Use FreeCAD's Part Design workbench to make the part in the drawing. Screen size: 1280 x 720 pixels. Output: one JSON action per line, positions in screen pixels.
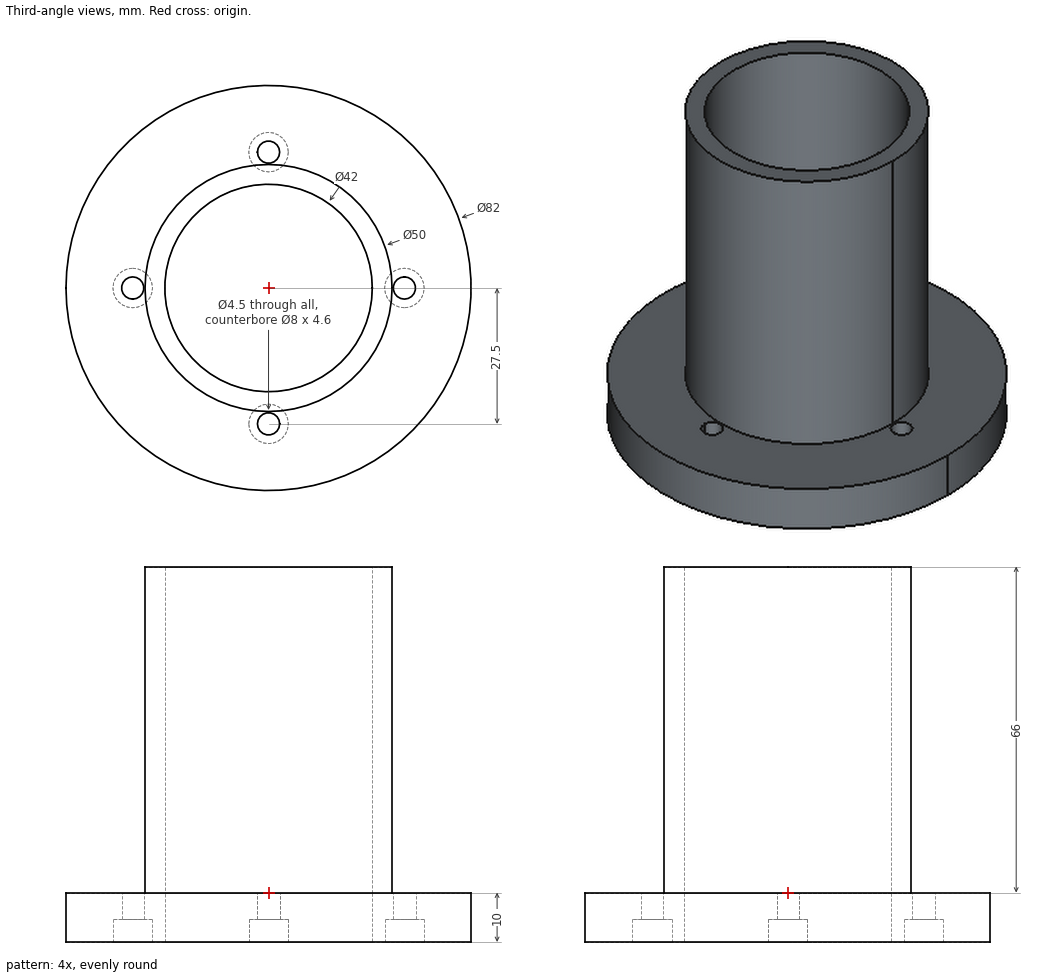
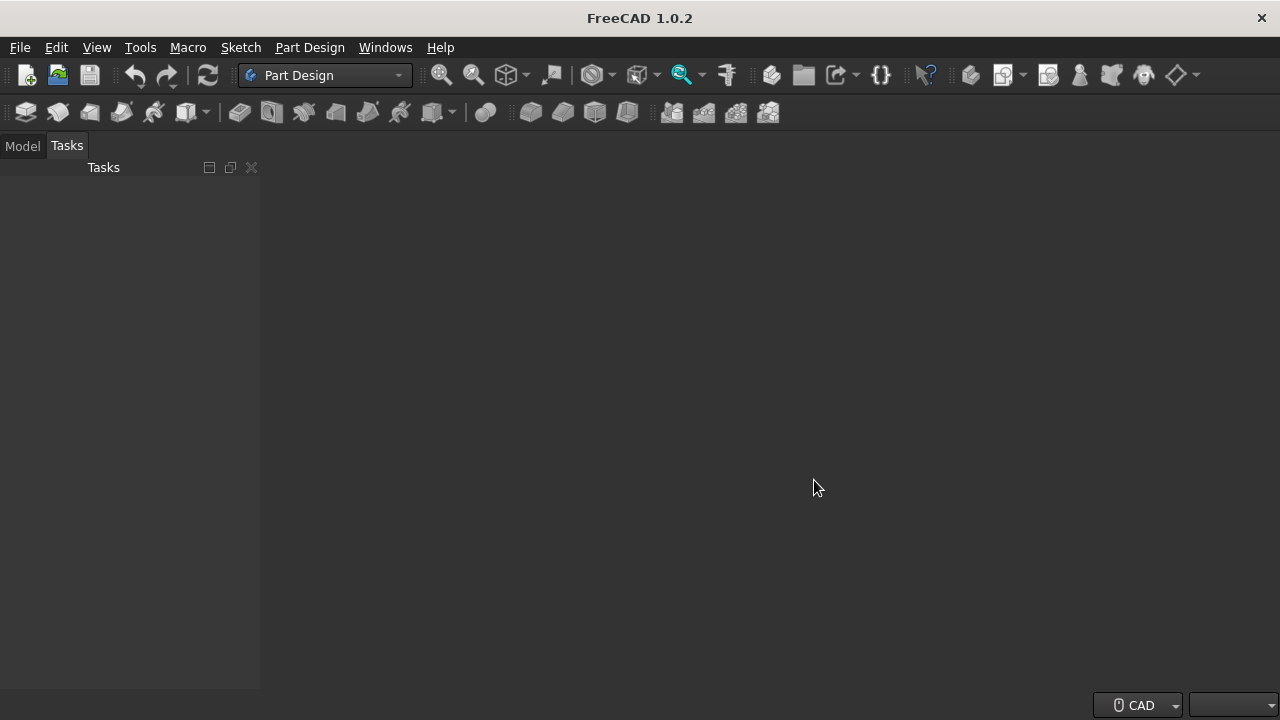
{"action": "left_click", "coordinate": [26, 76]}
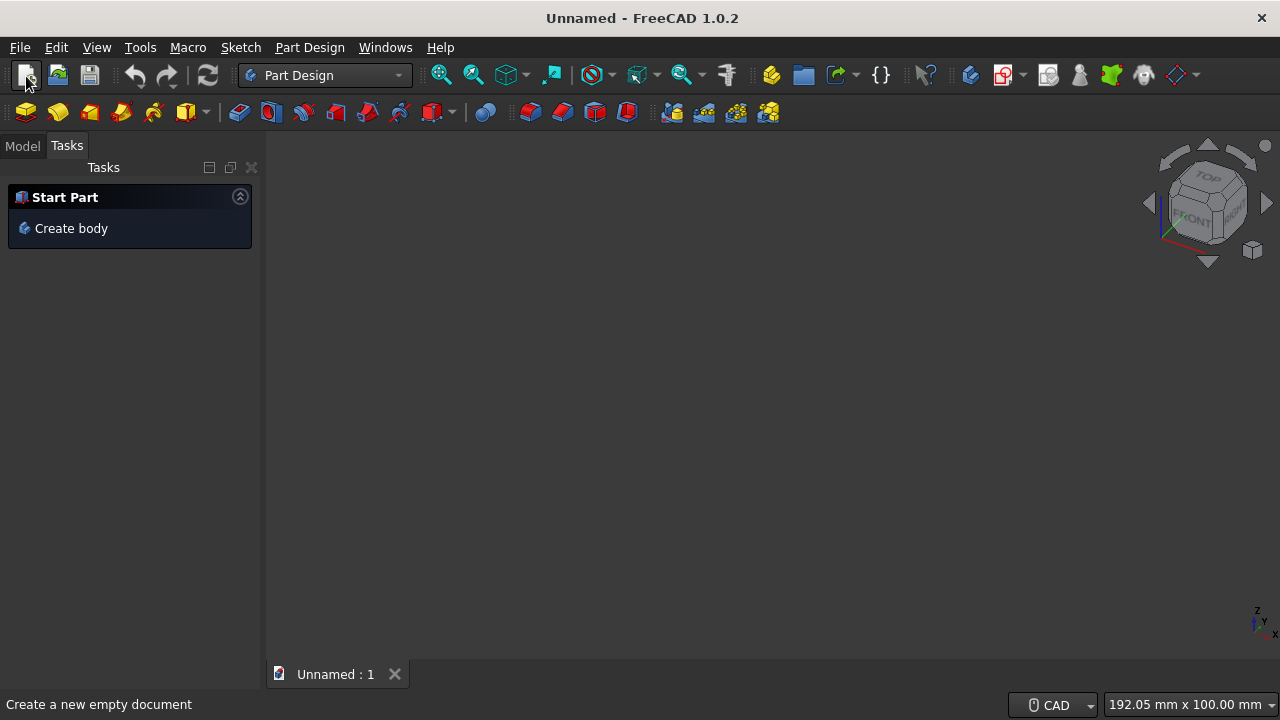
{"action": "left_click", "coordinate": [1004, 76]}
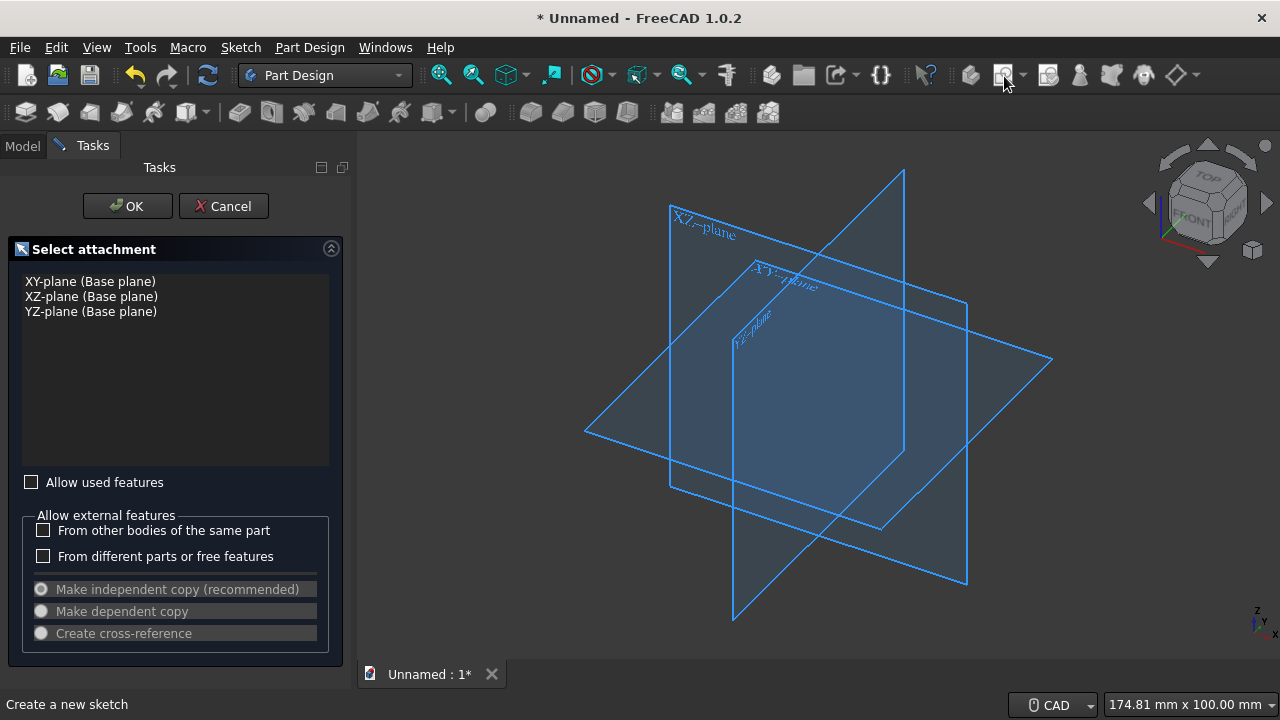
{"action": "left_click", "coordinate": [82, 282]}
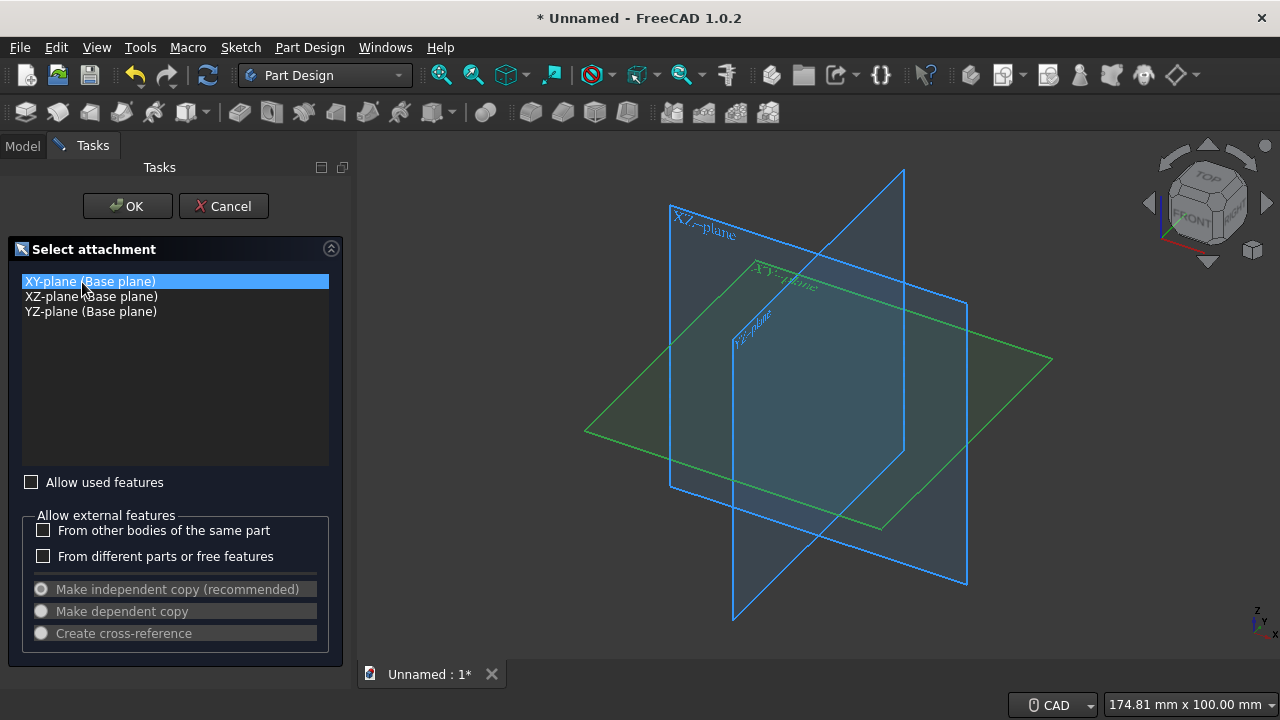
{"action": "left_click", "coordinate": [128, 206]}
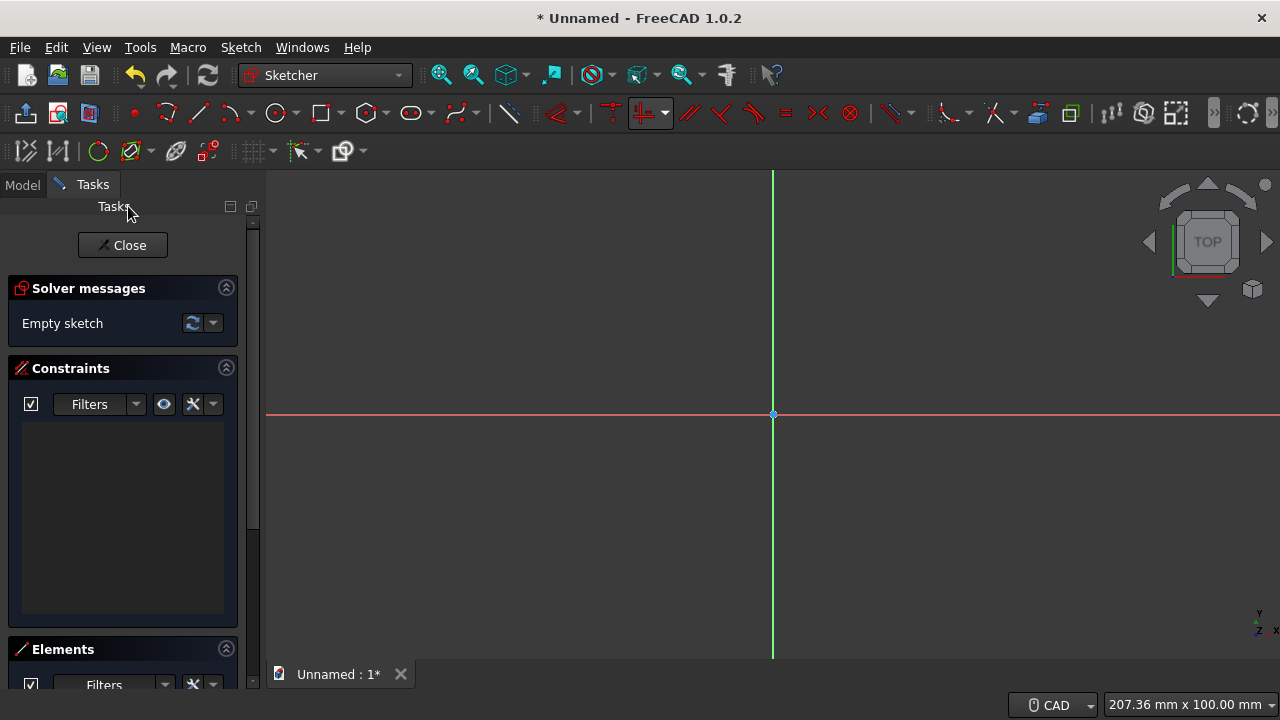
{"action": "key", "text": "g c"}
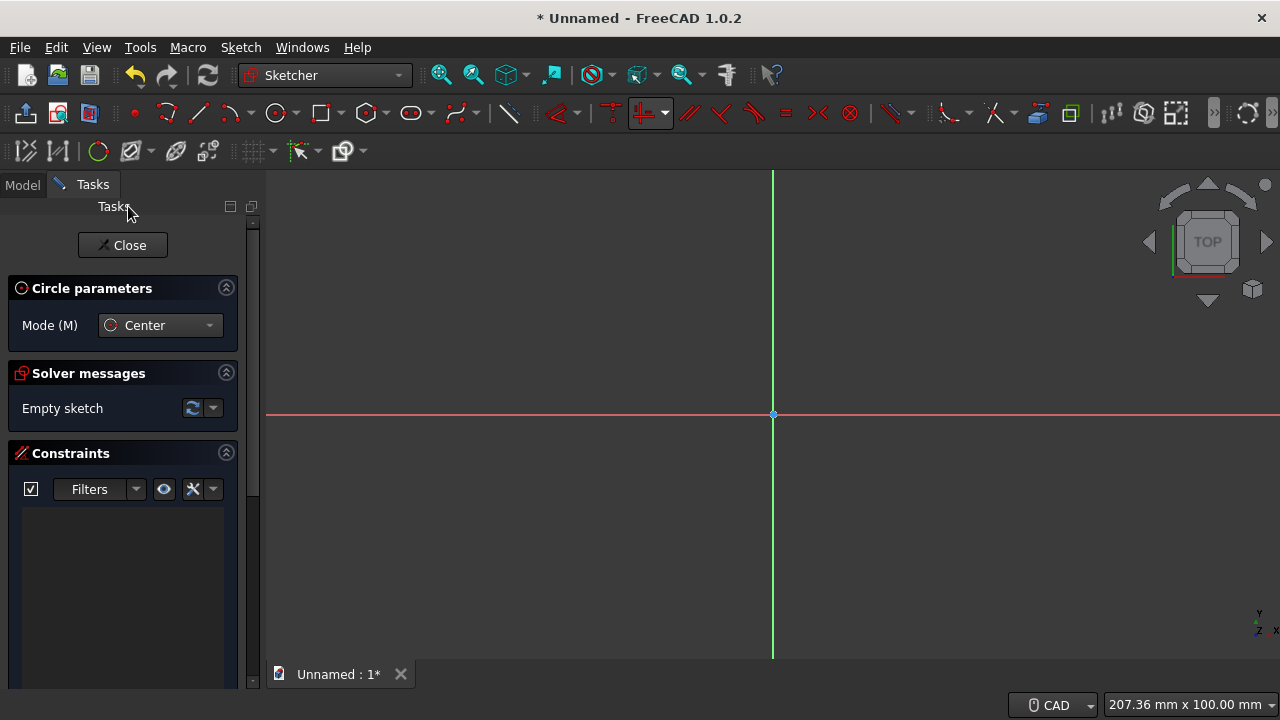
{"action": "left_click", "coordinate": [773, 414]}
{"action": "left_click", "coordinate": [859, 328]}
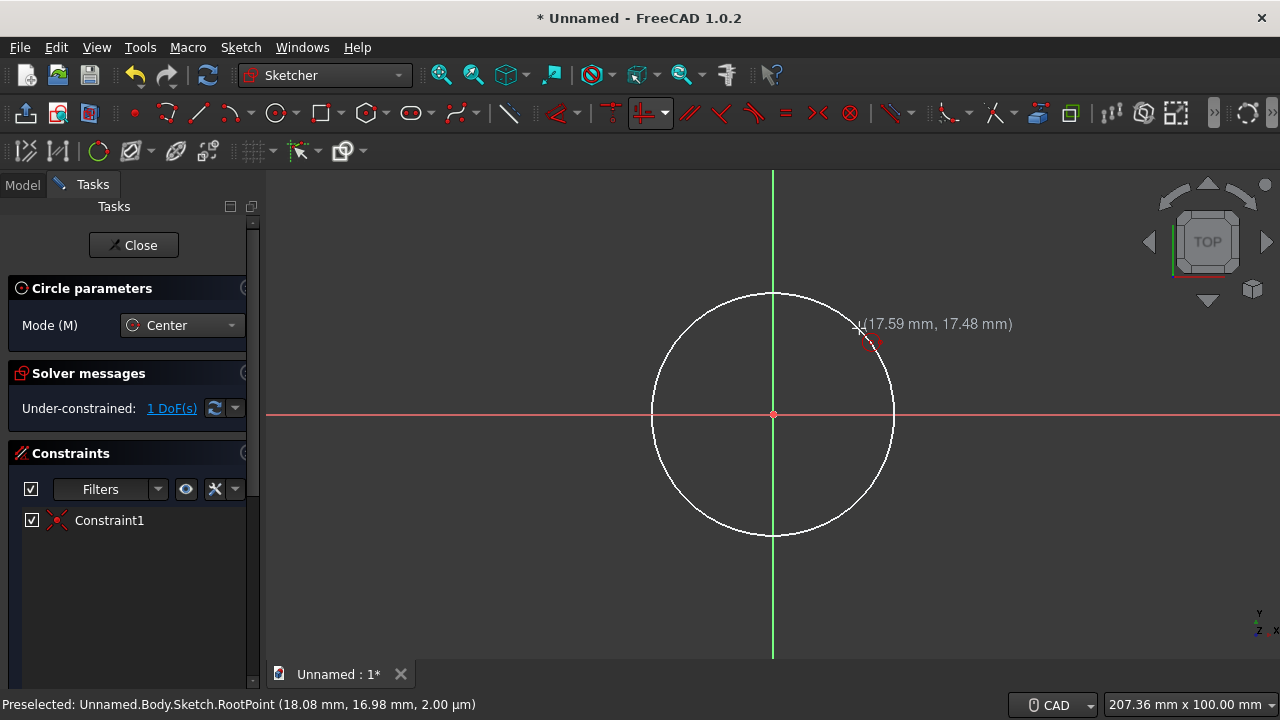
{"action": "left_click", "coordinate": [773, 414]}
{"action": "left_click", "coordinate": [846, 342]}
{"action": "key", "text": "Escape"}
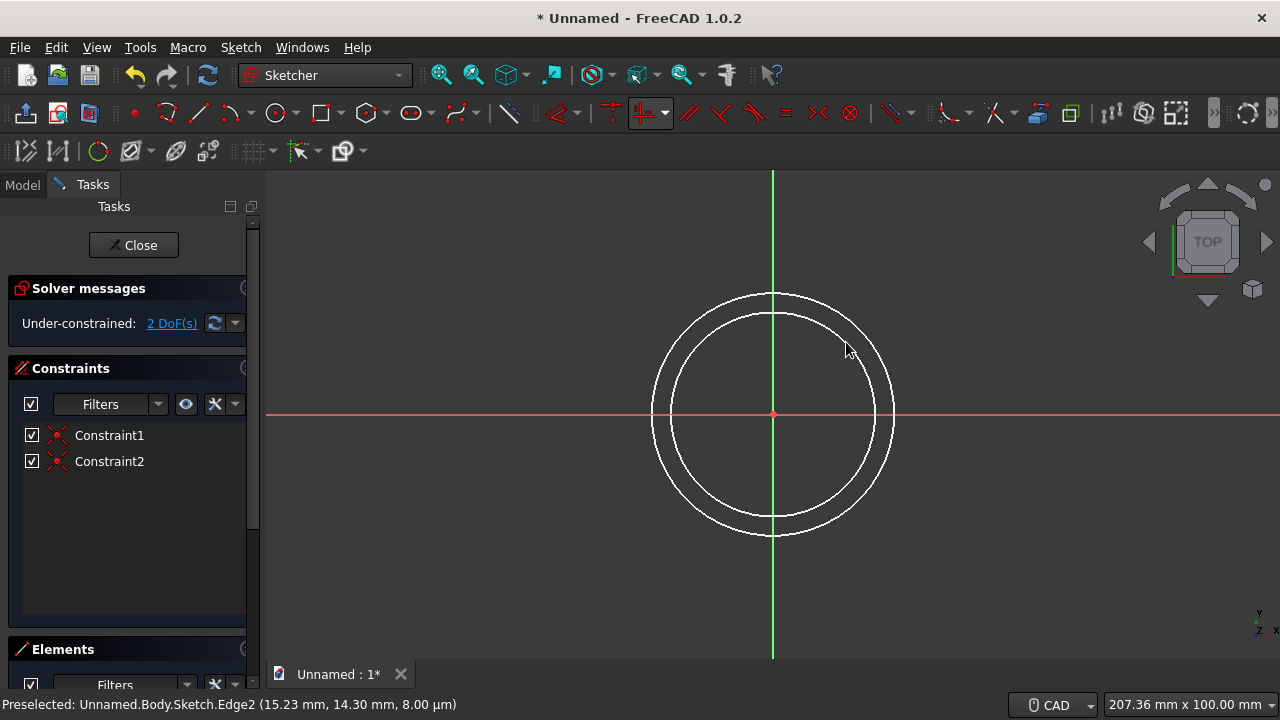
{"action": "left_click", "coordinate": [556, 114]}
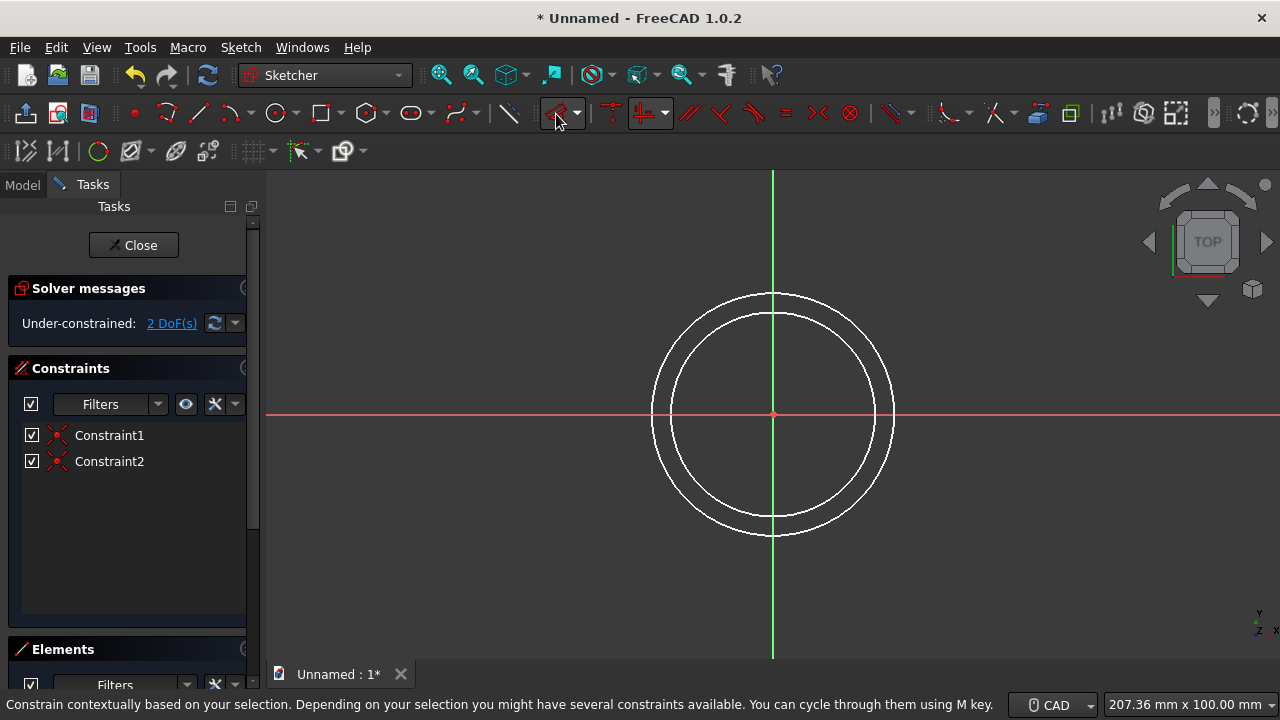
{"action": "left_click", "coordinate": [858, 328]}
{"action": "left_click", "coordinate": [880, 305]}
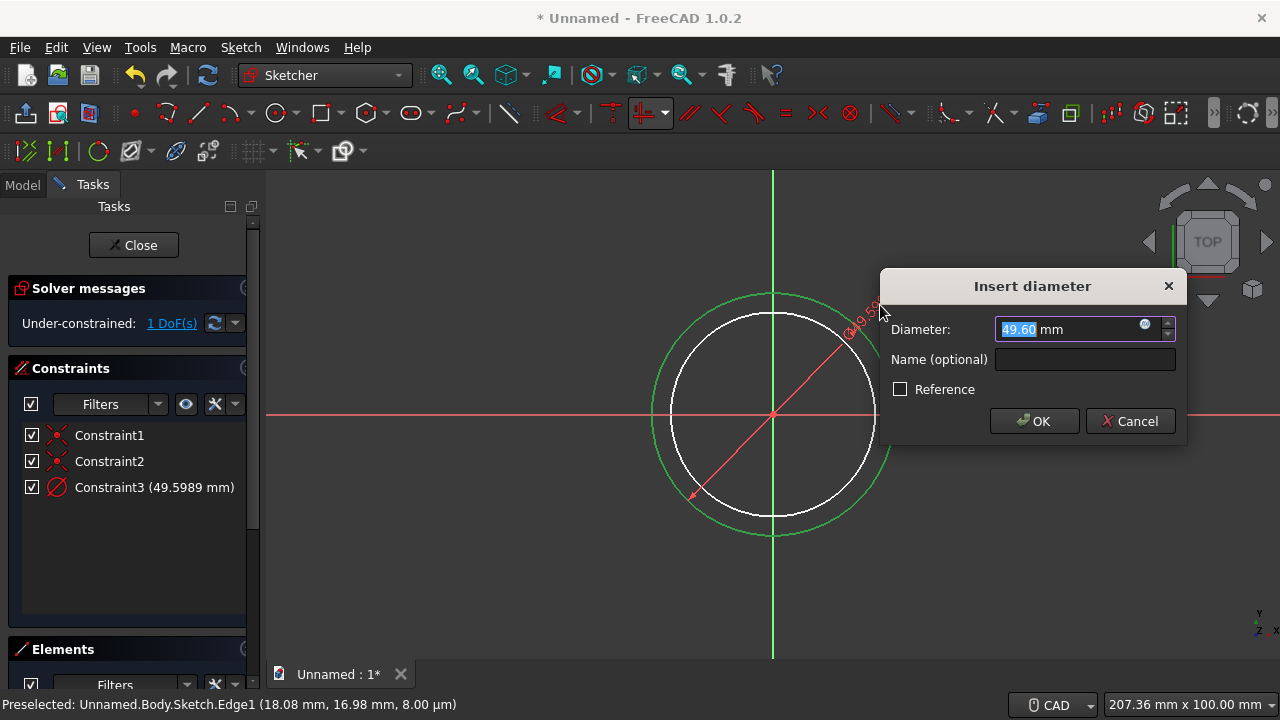
{"action": "type", "text": "50"}
{"action": "key", "text": "Return"}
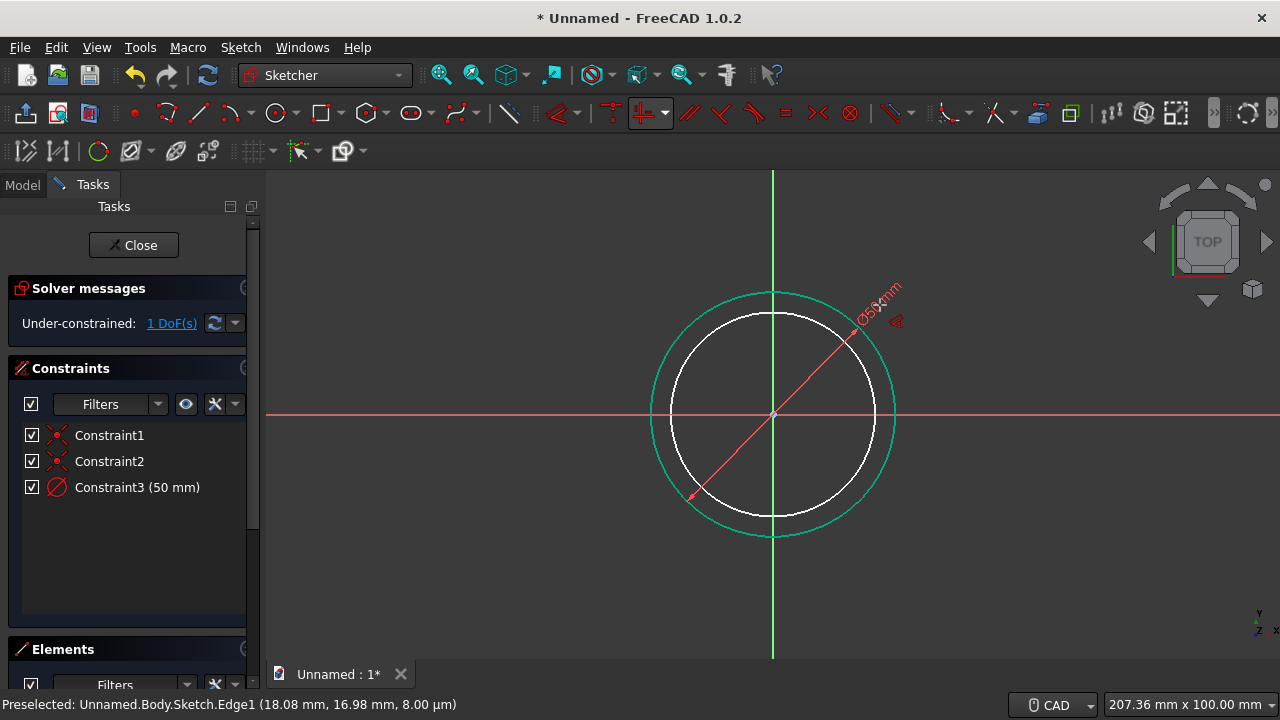
{"action": "left_click", "coordinate": [845, 342]}
{"action": "left_click", "coordinate": [924, 370]}